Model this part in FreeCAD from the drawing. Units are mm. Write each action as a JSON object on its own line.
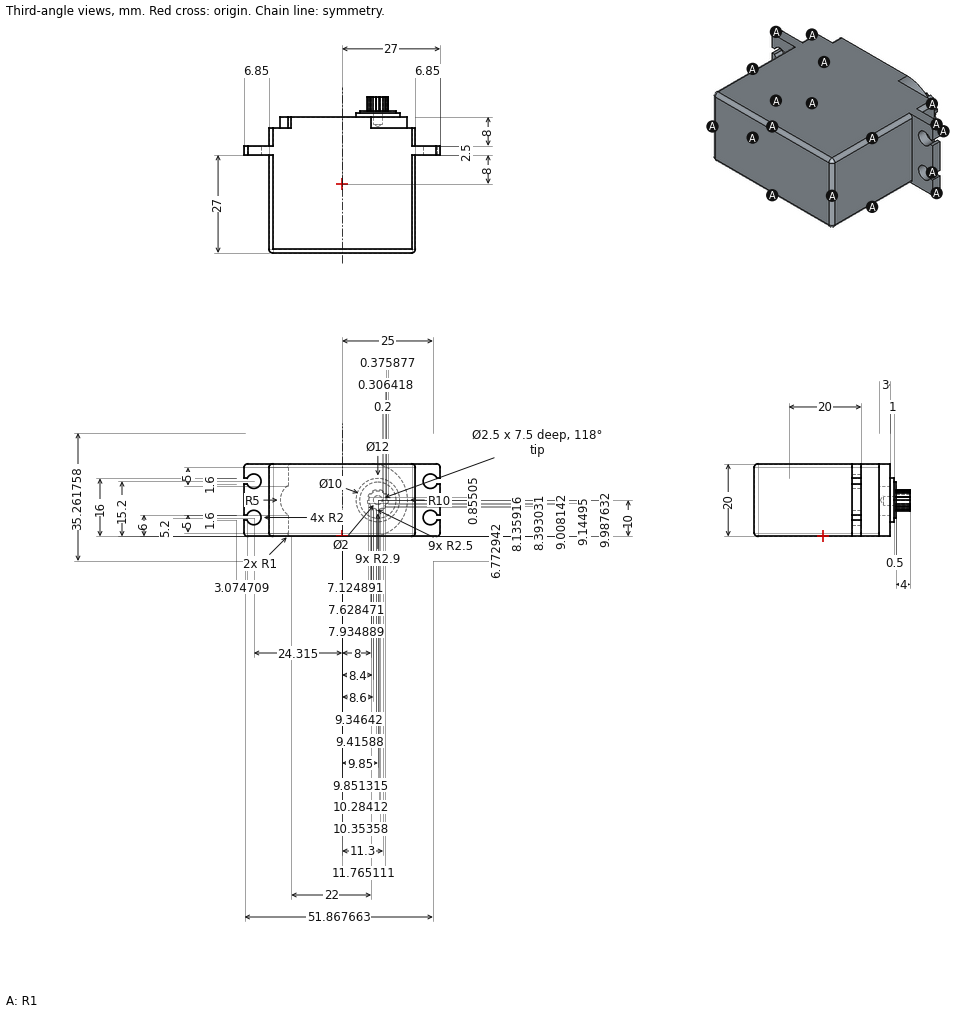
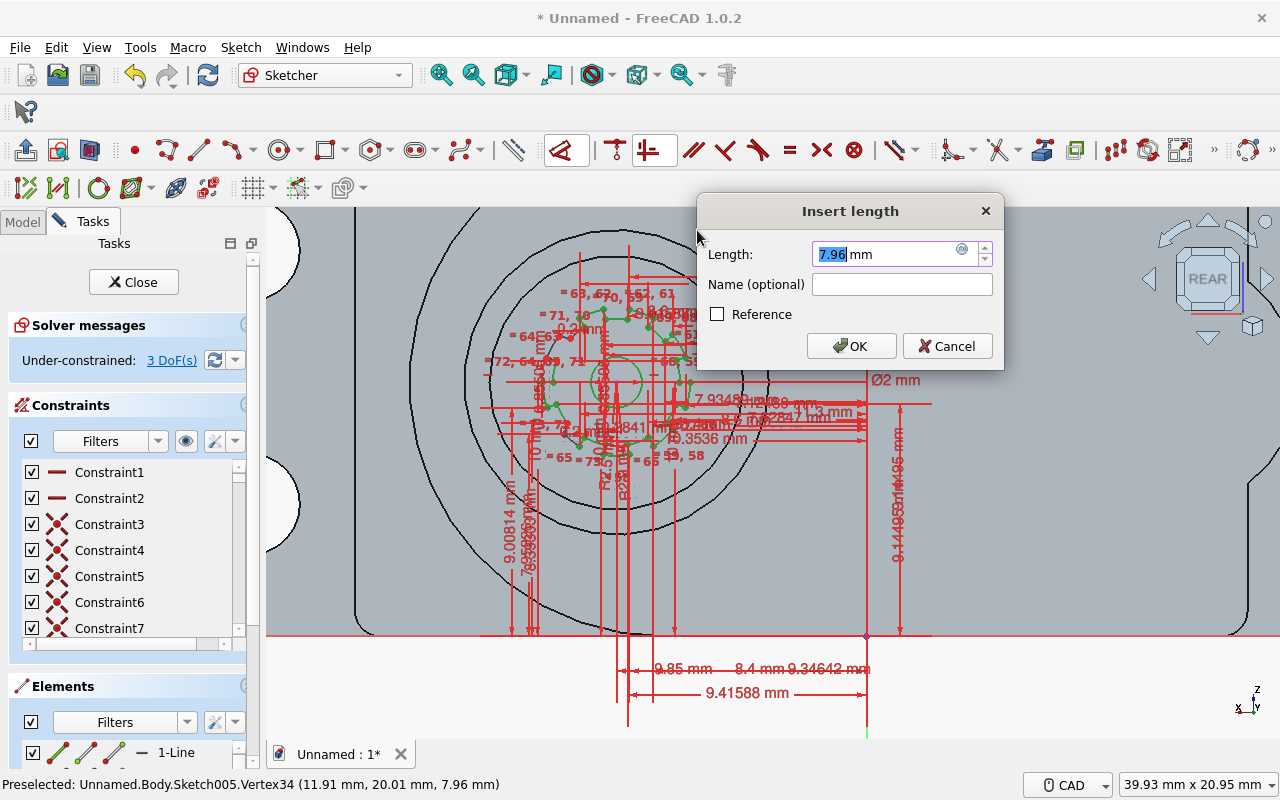
{"action": "type", "text": "8.135916"}
{"action": "key", "text": "Return"}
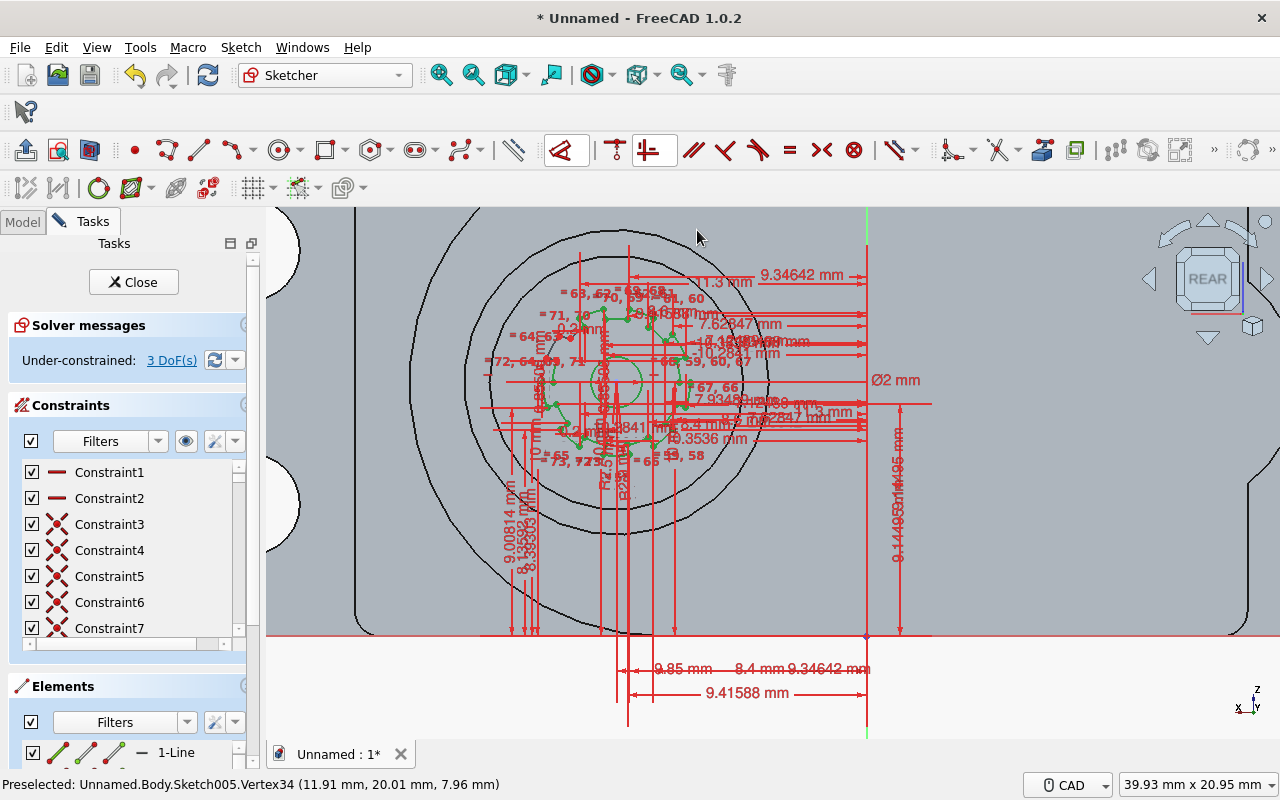
{"action": "scroll", "coordinate": [565, 337], "scroll_direction": "up", "scroll_amount": 9}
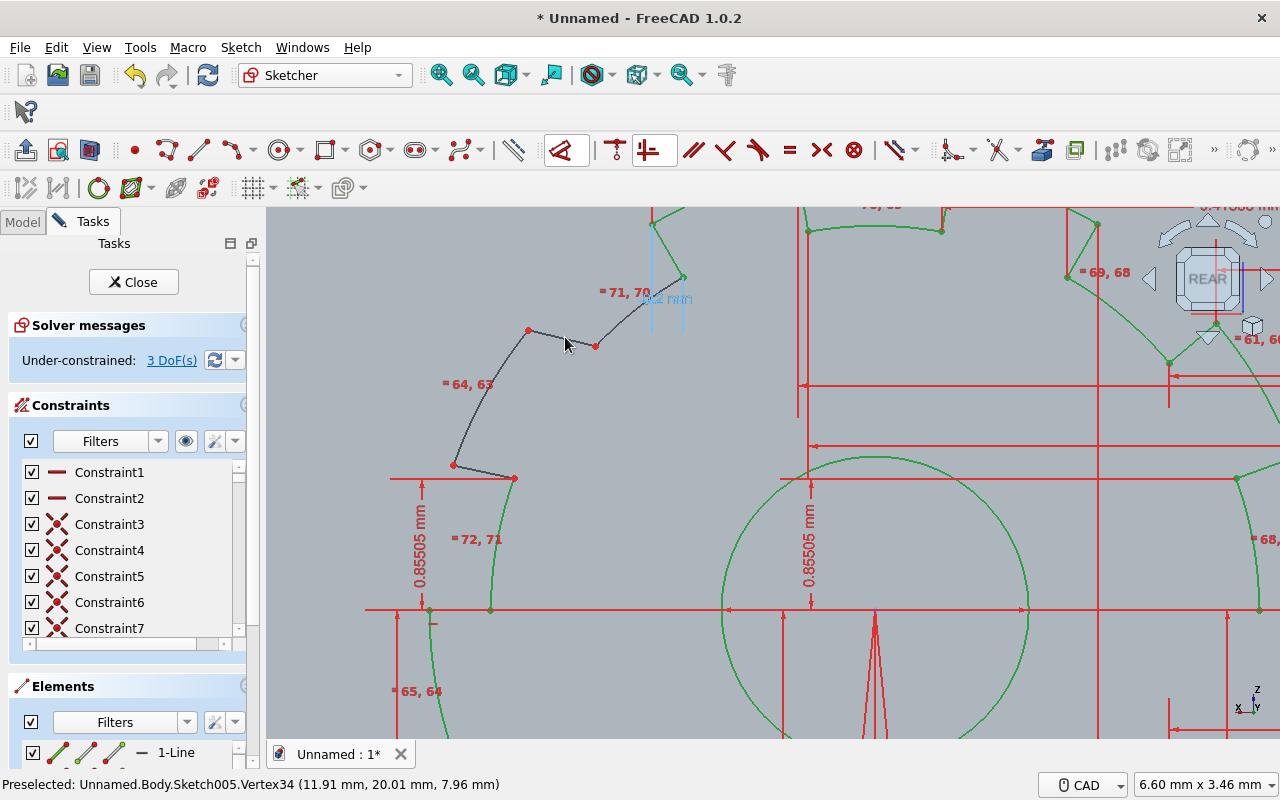
{"action": "left_click", "coordinate": [562, 338]}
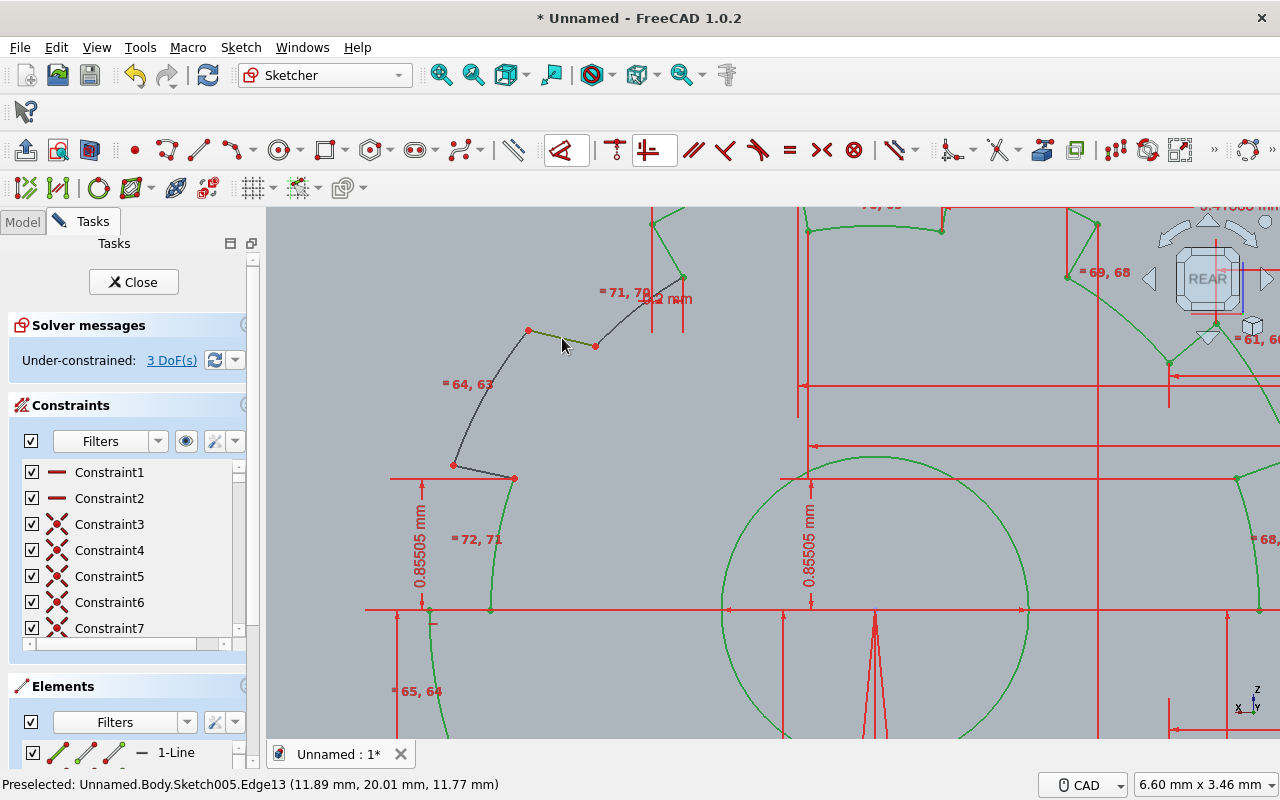
{"action": "key", "text": "l"}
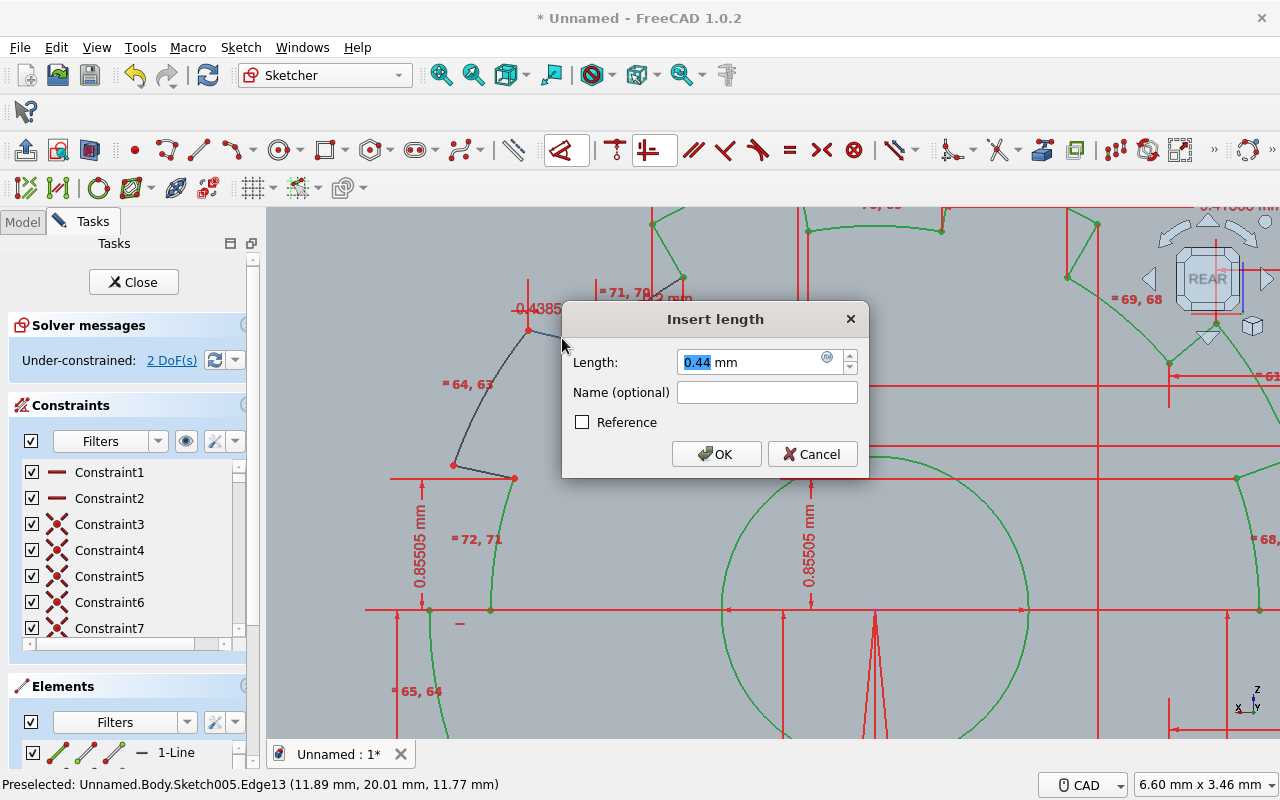
{"action": "type", "text": "0.306418"}
{"action": "key", "text": "Return"}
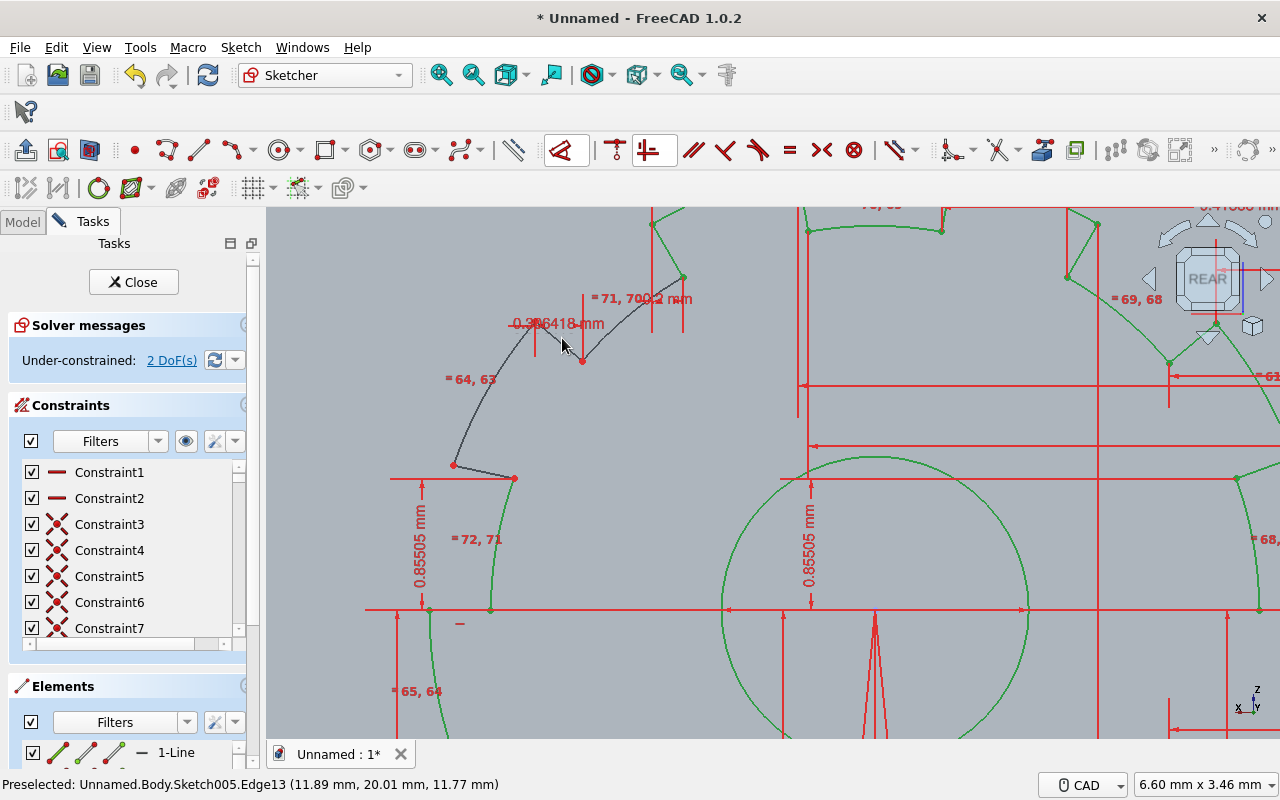
{"action": "left_click", "coordinate": [472, 470]}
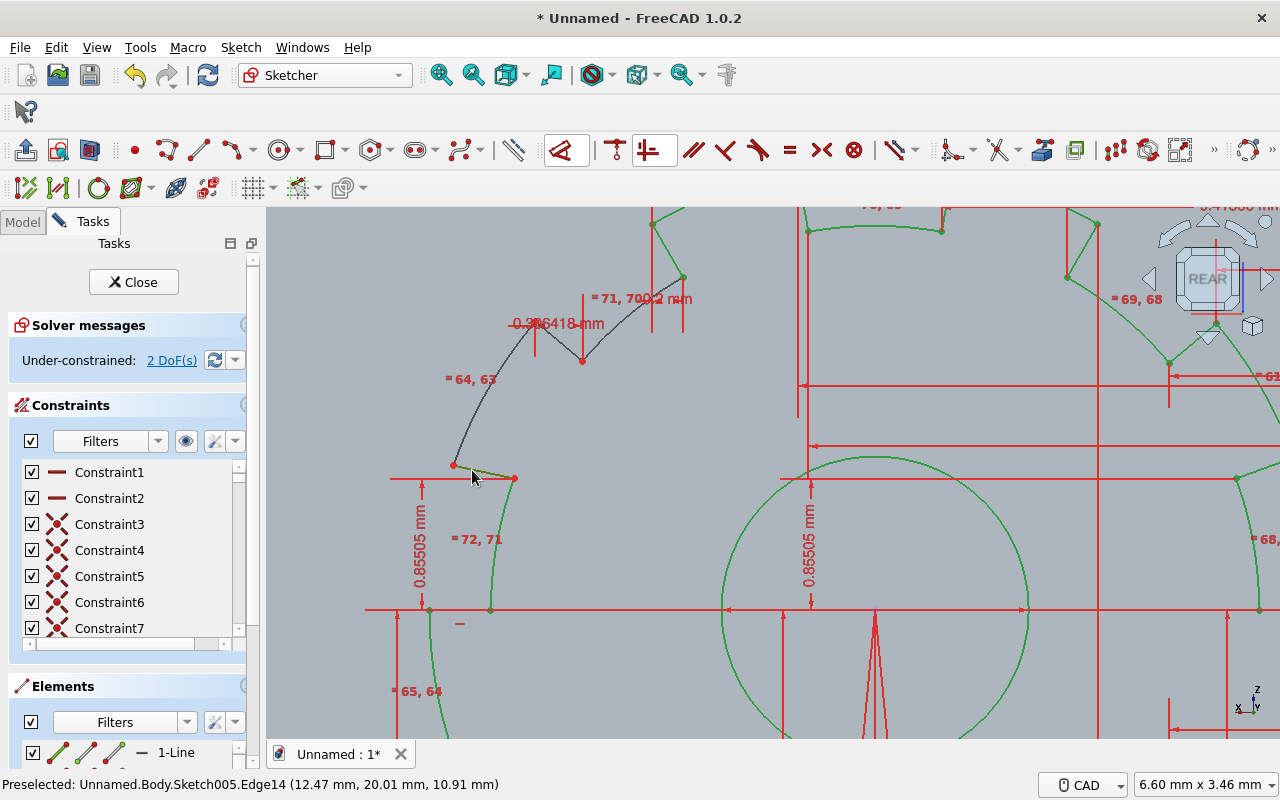
{"action": "key", "text": "l"}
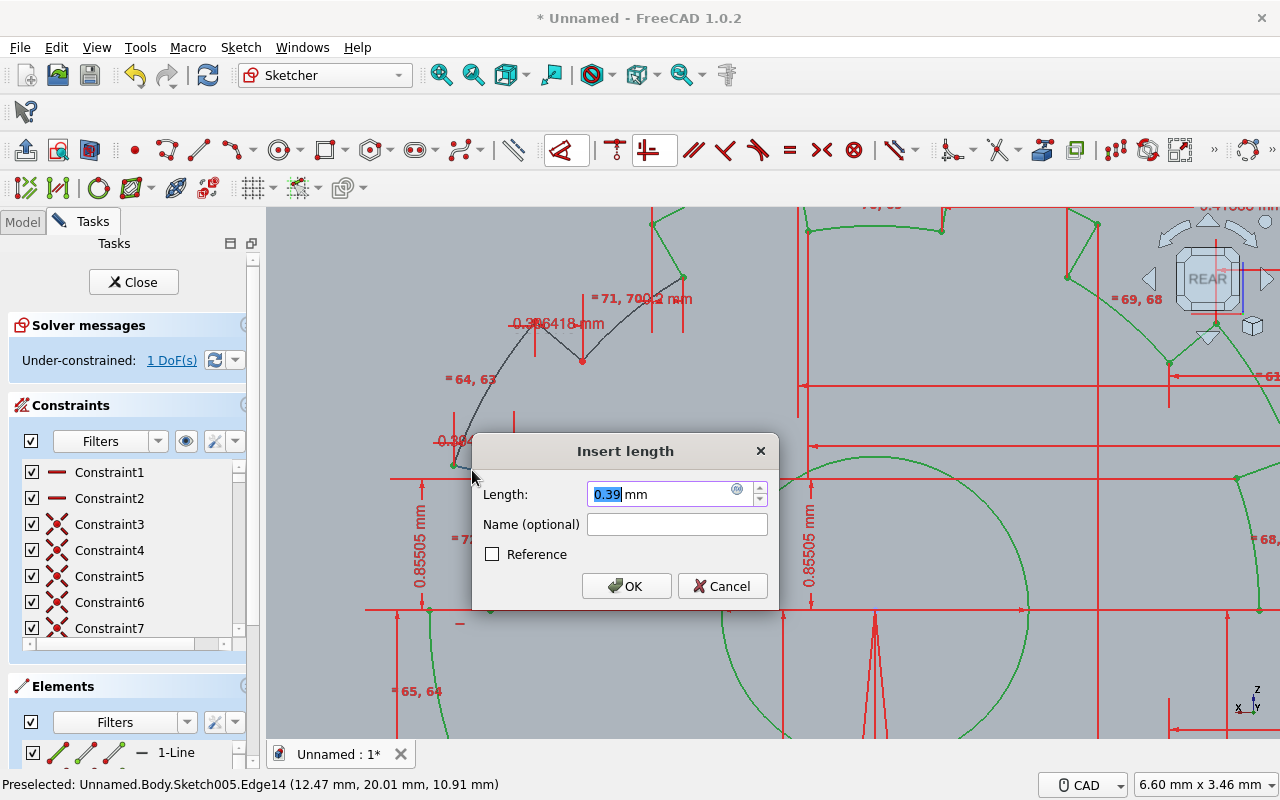
{"action": "type", "text": "0.375877"}
{"action": "key", "text": "Return"}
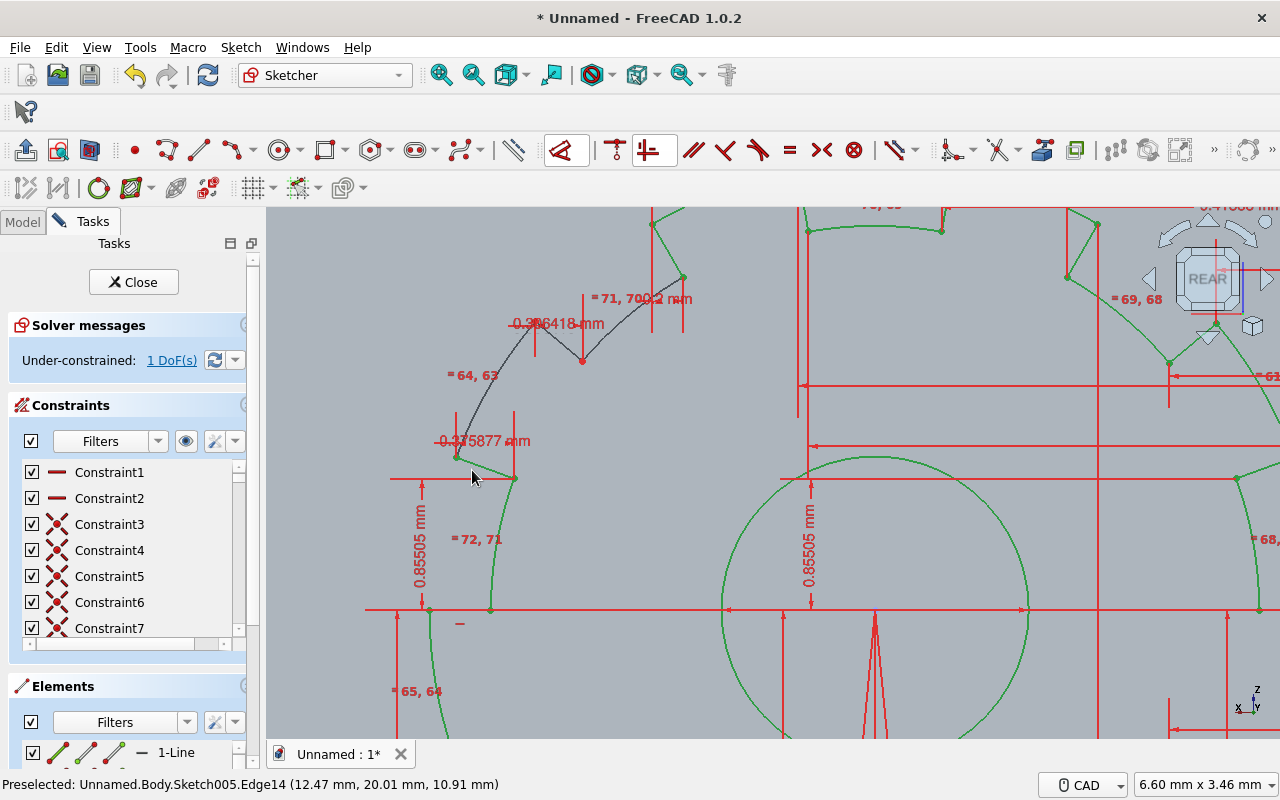
{"action": "scroll", "coordinate": [565, 337], "scroll_direction": "down", "scroll_amount": 9}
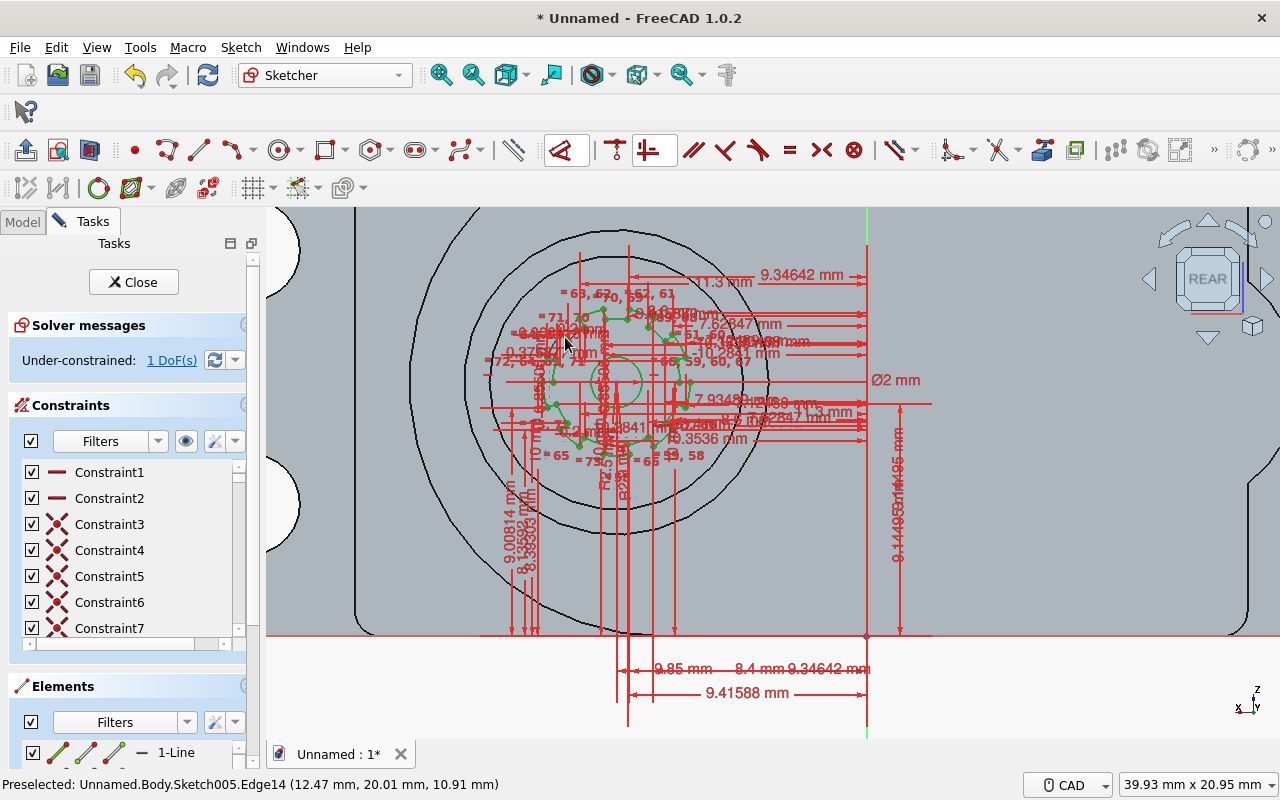
{"action": "left_click", "coordinate": [568, 341]}